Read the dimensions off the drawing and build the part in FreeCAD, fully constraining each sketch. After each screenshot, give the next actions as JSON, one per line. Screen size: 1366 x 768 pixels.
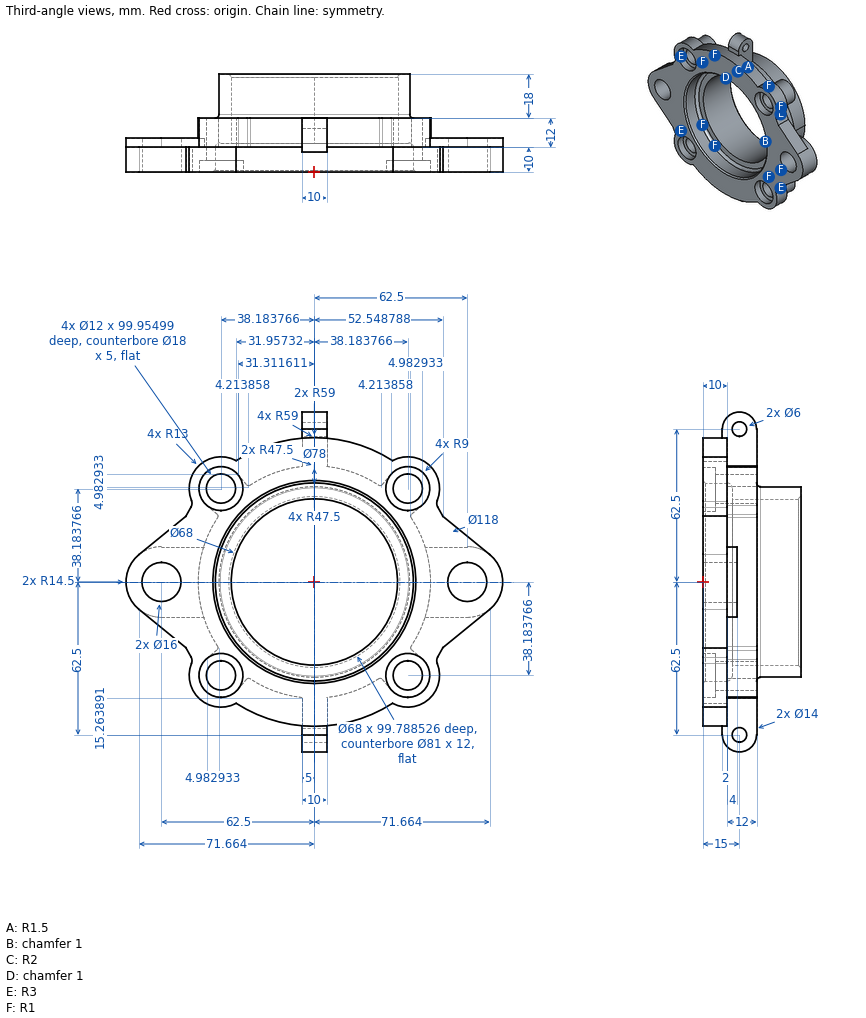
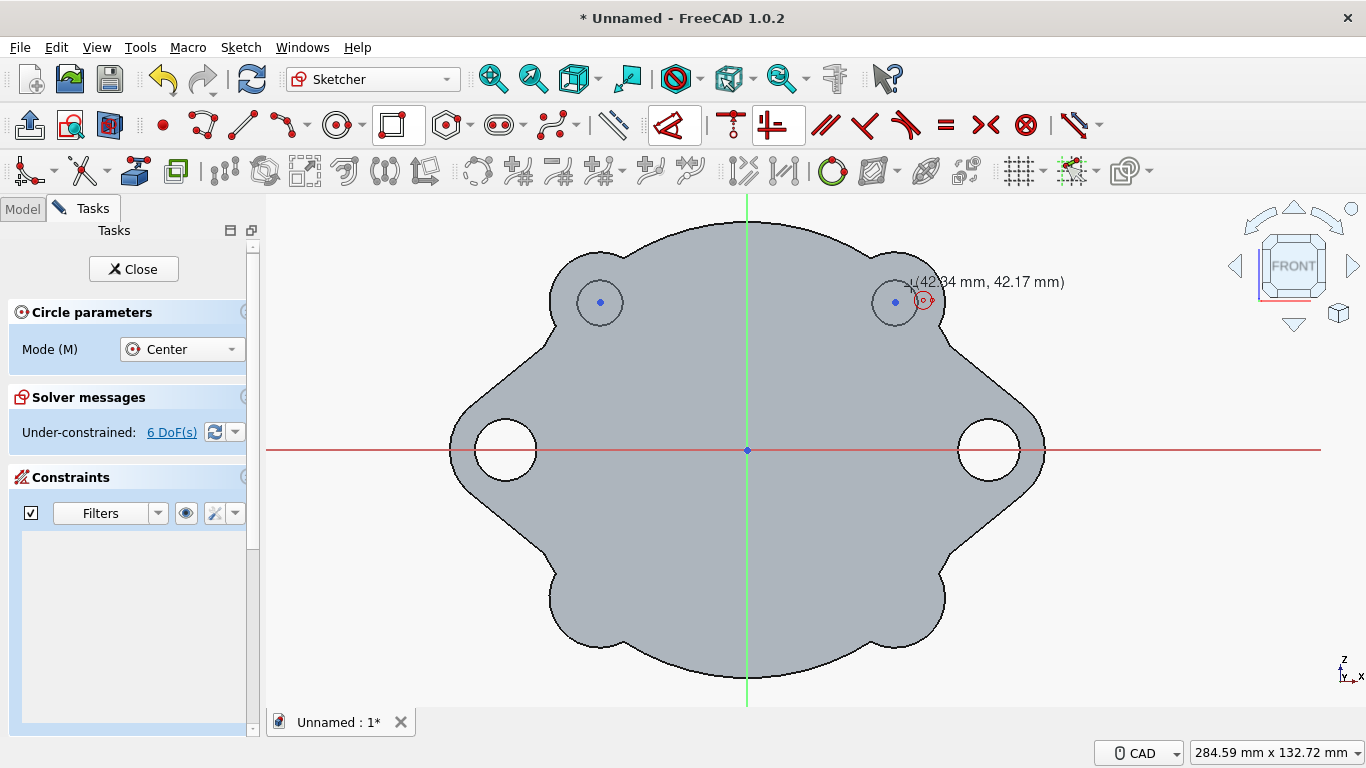
{"action": "left_click", "coordinate": [895, 598]}
{"action": "left_click", "coordinate": [911, 581]}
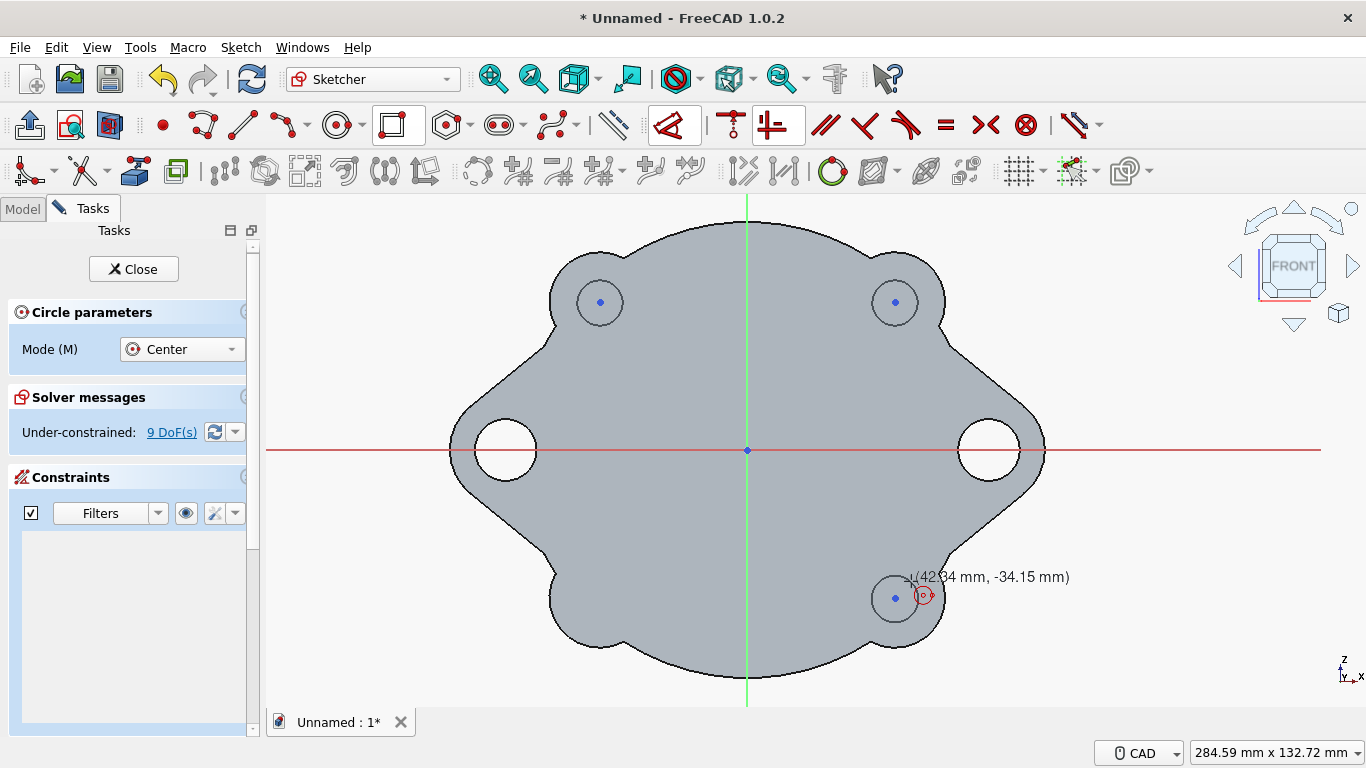
{"action": "left_click", "coordinate": [600, 598]}
{"action": "left_click", "coordinate": [616, 581]}
{"action": "key", "text": "Escape"}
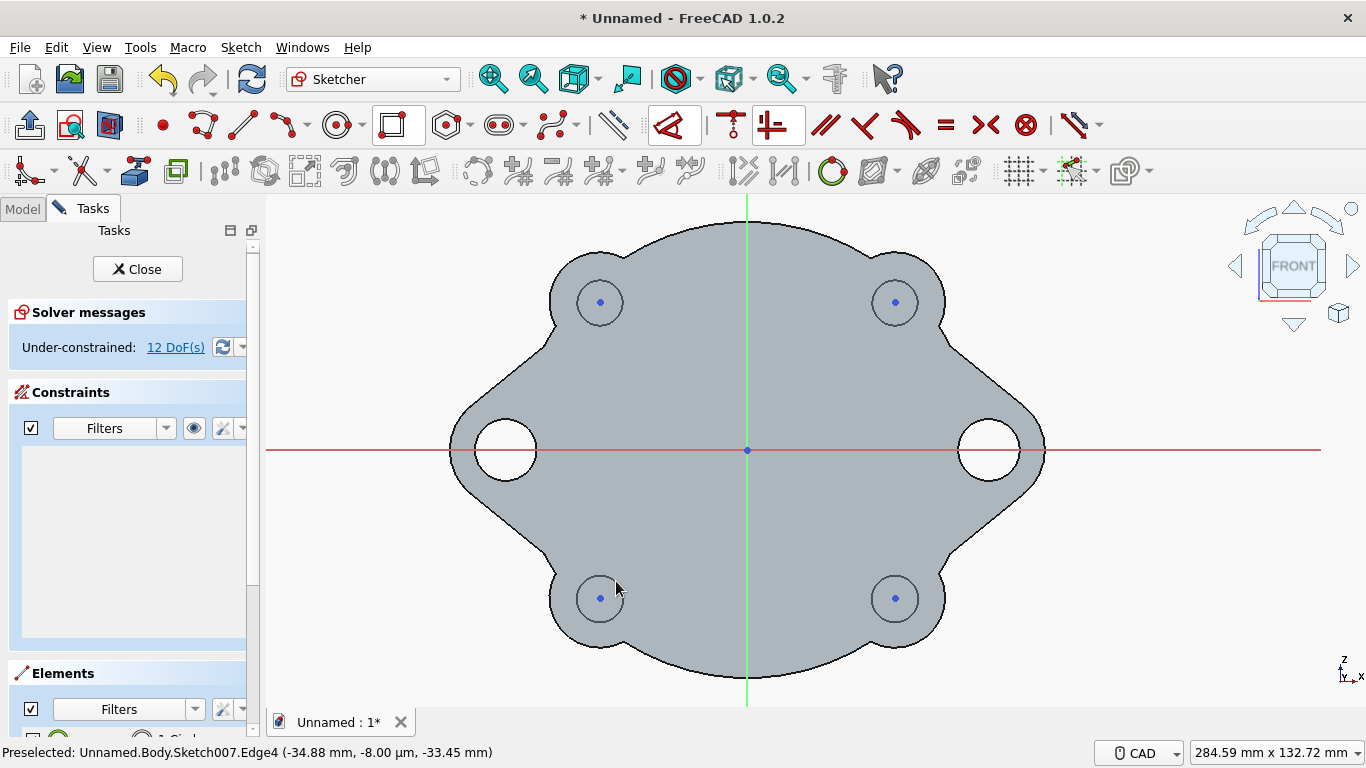
{"action": "left_click", "coordinate": [616, 287]}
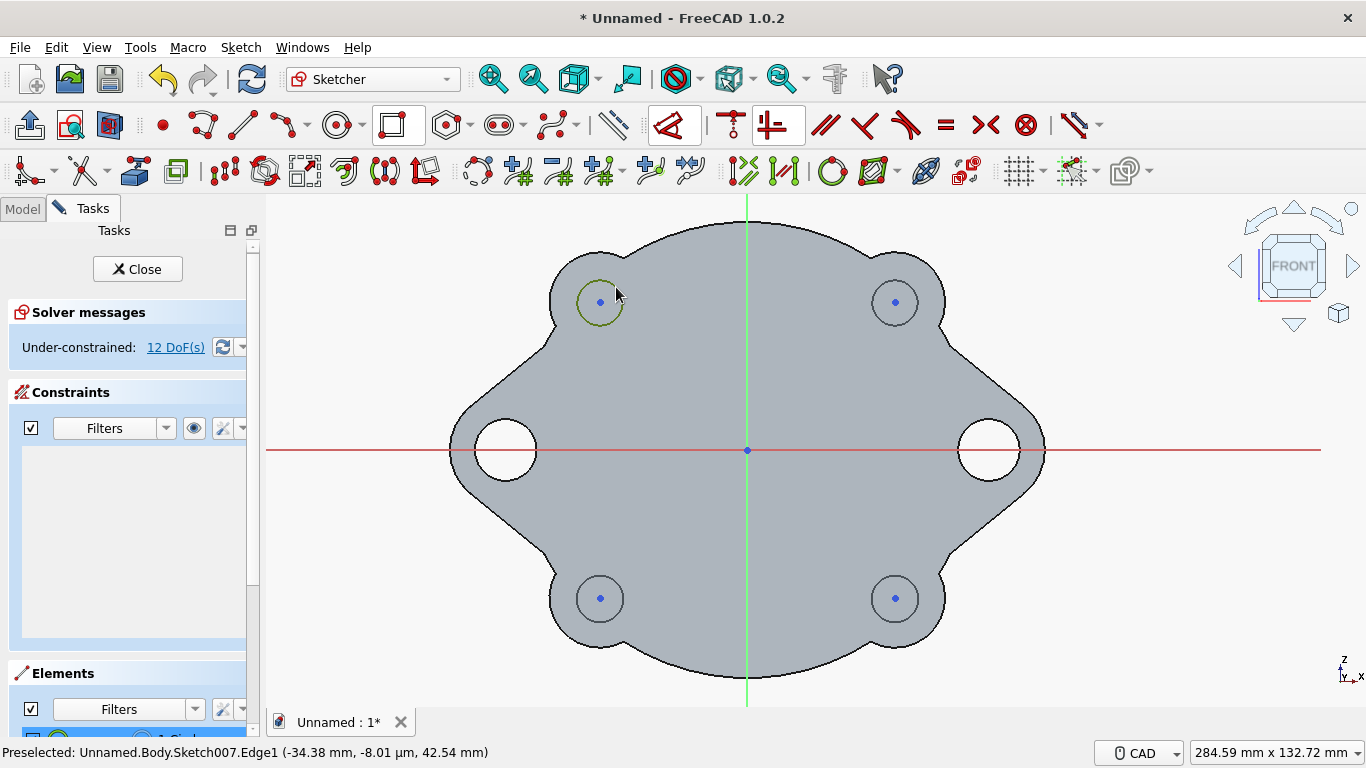
{"action": "left_click", "coordinate": [911, 287]}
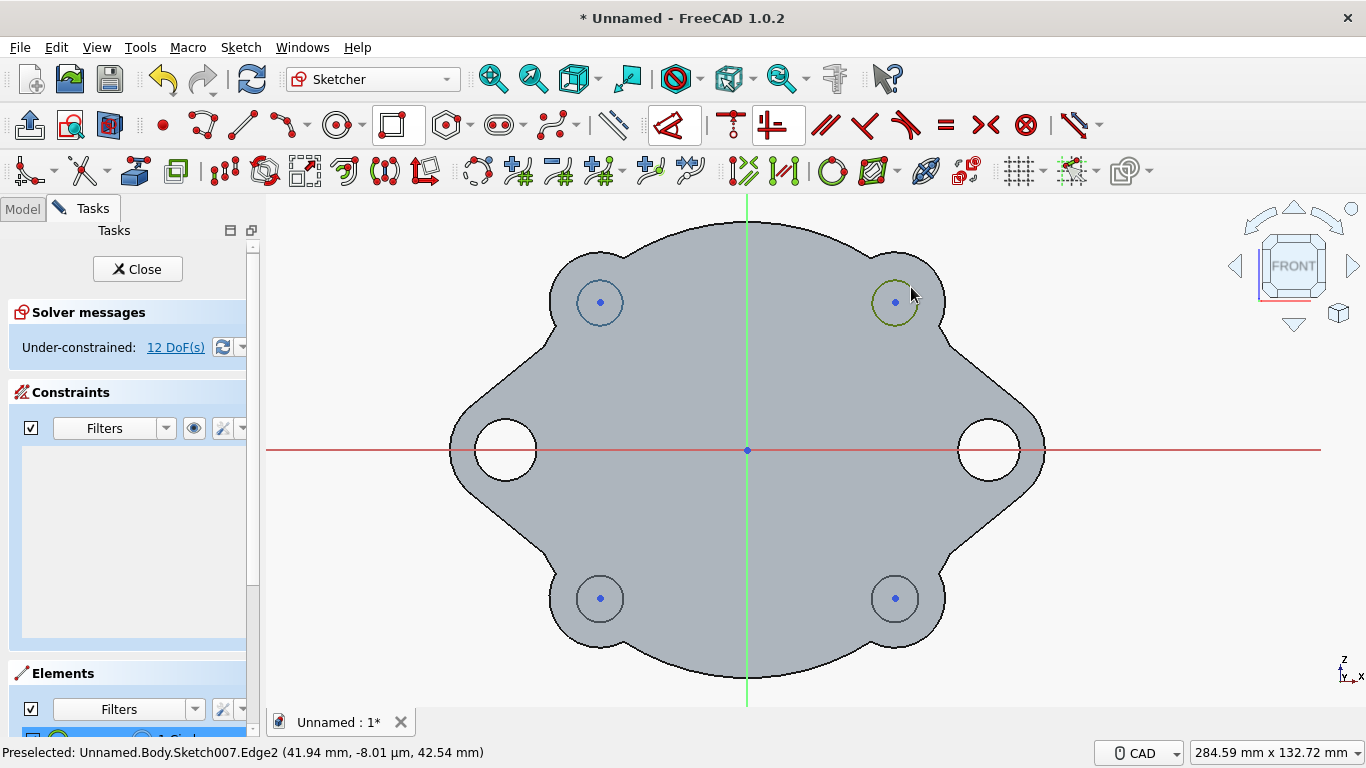
{"action": "left_click", "coordinate": [911, 582]}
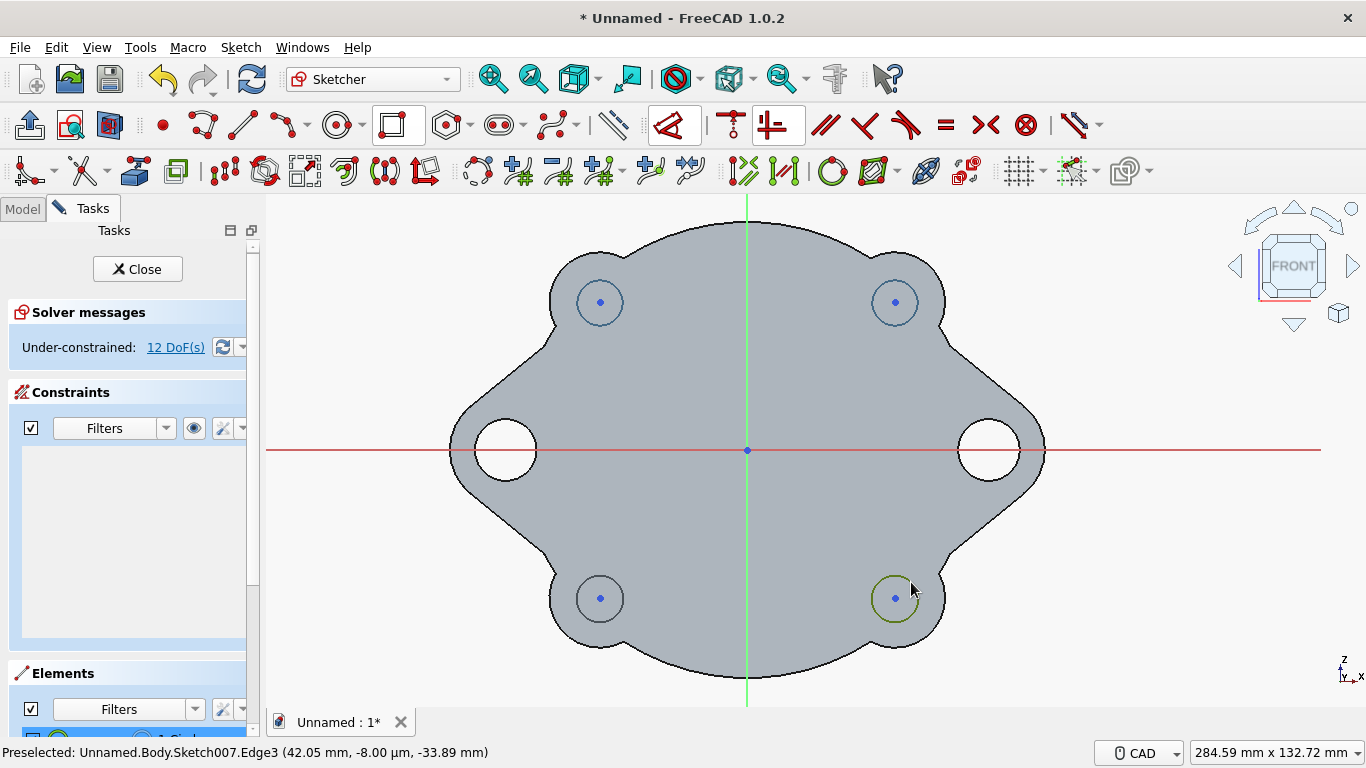
{"action": "left_click", "coordinate": [616, 582]}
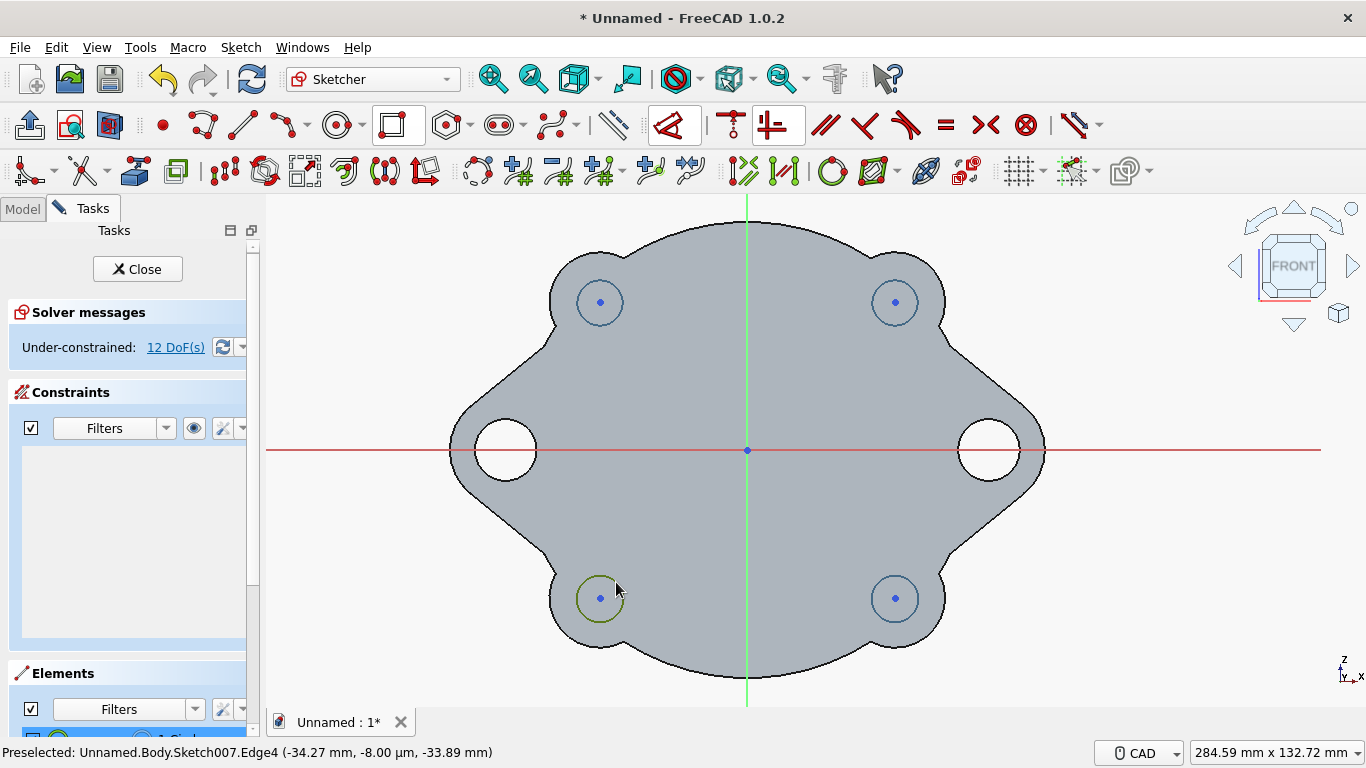
{"action": "left_click", "coordinate": [946, 126]}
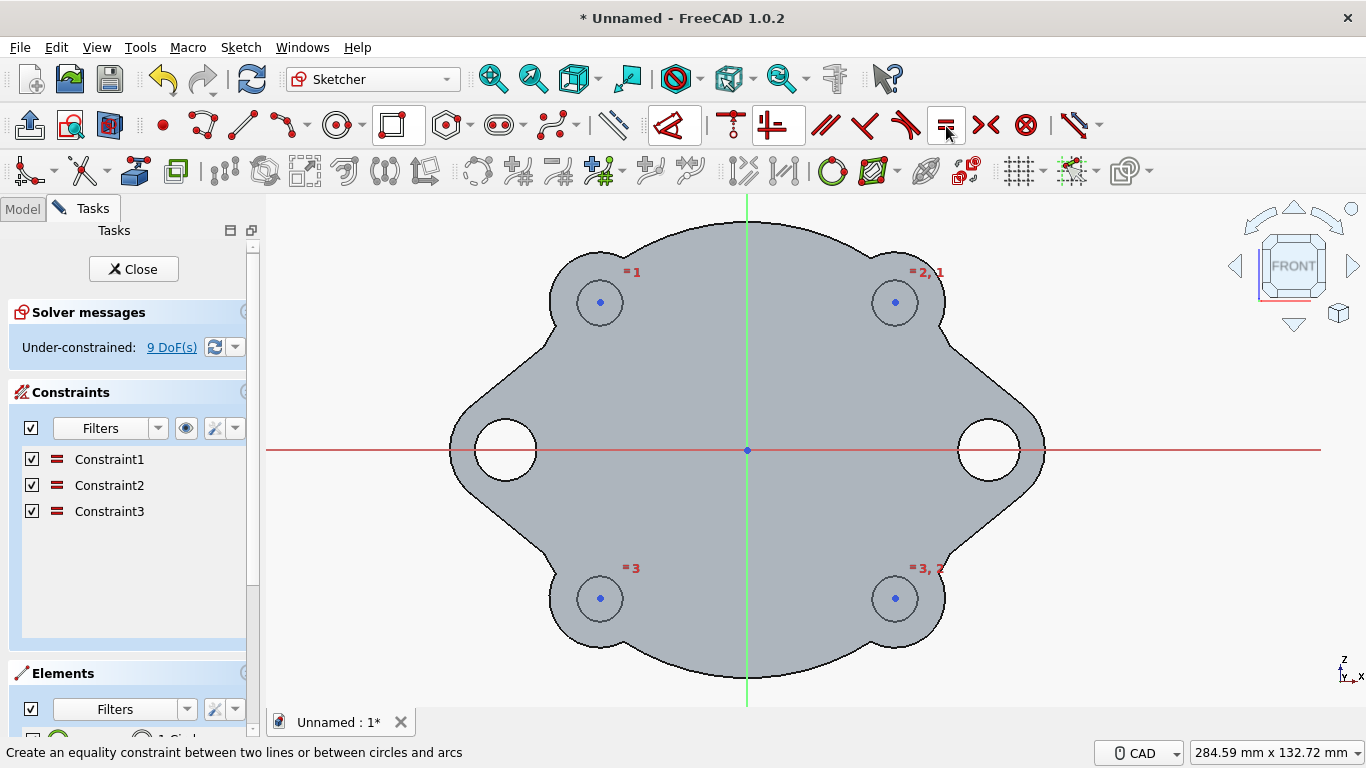
{"action": "left_click", "coordinate": [600, 303]}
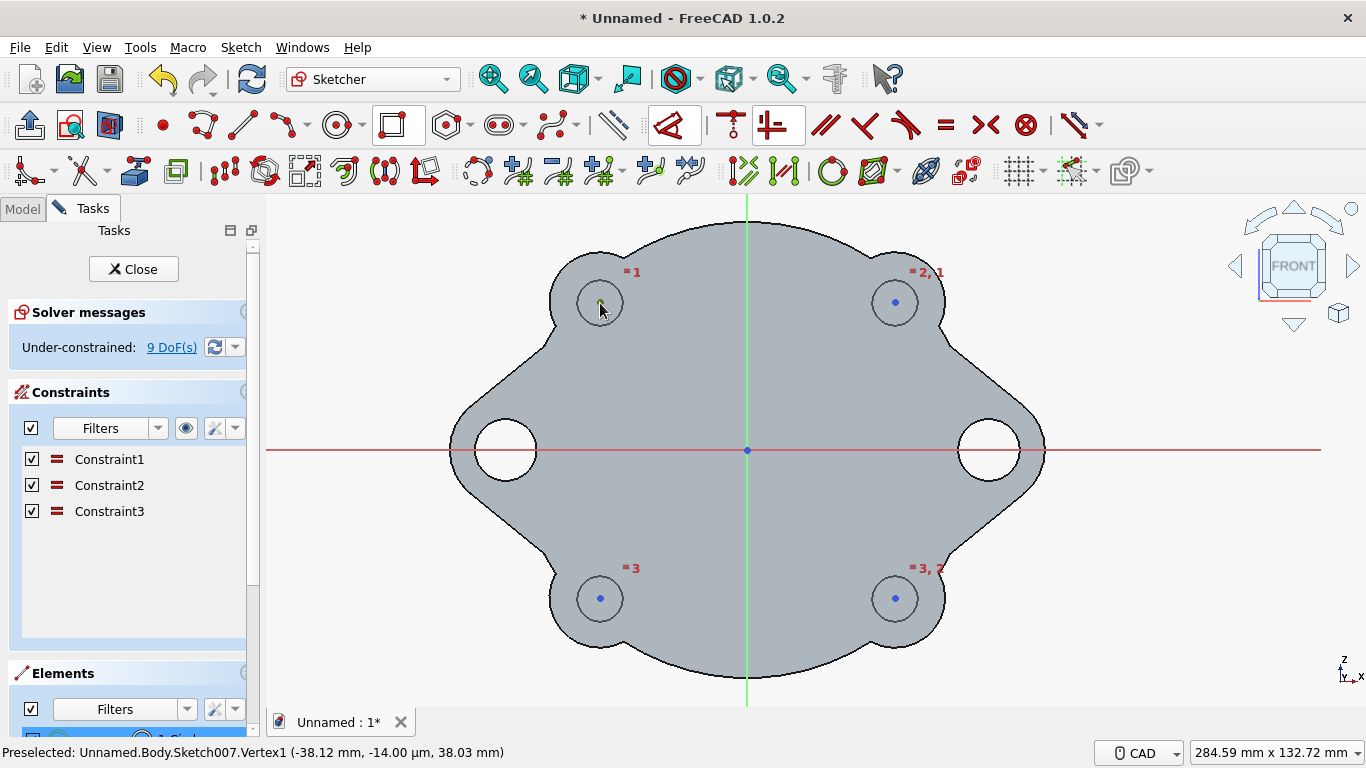
{"action": "left_click", "coordinate": [895, 303]}